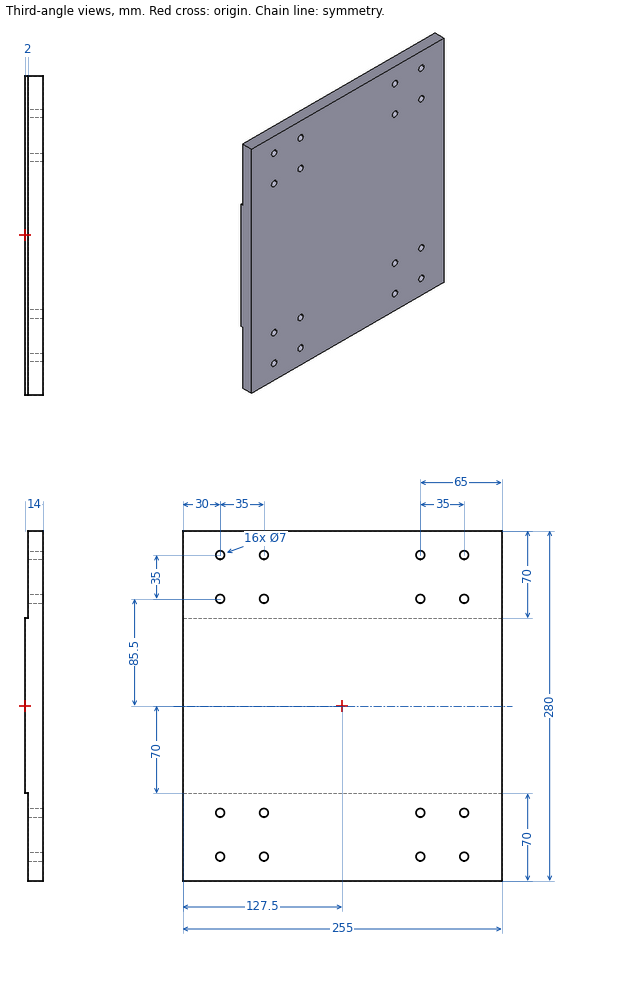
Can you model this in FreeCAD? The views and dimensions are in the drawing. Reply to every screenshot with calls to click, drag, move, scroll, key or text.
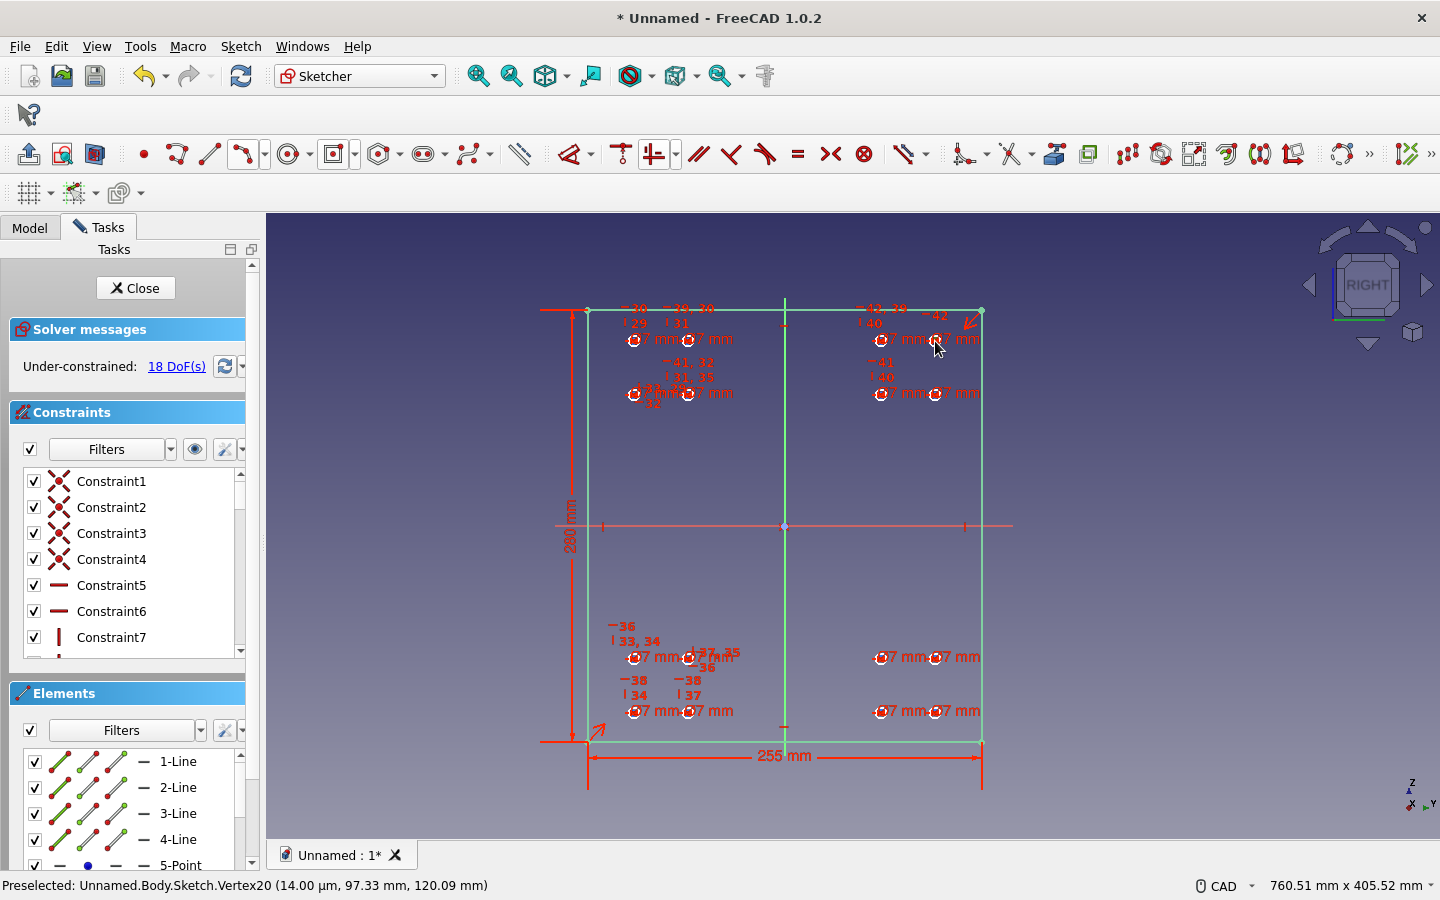
click(935, 395)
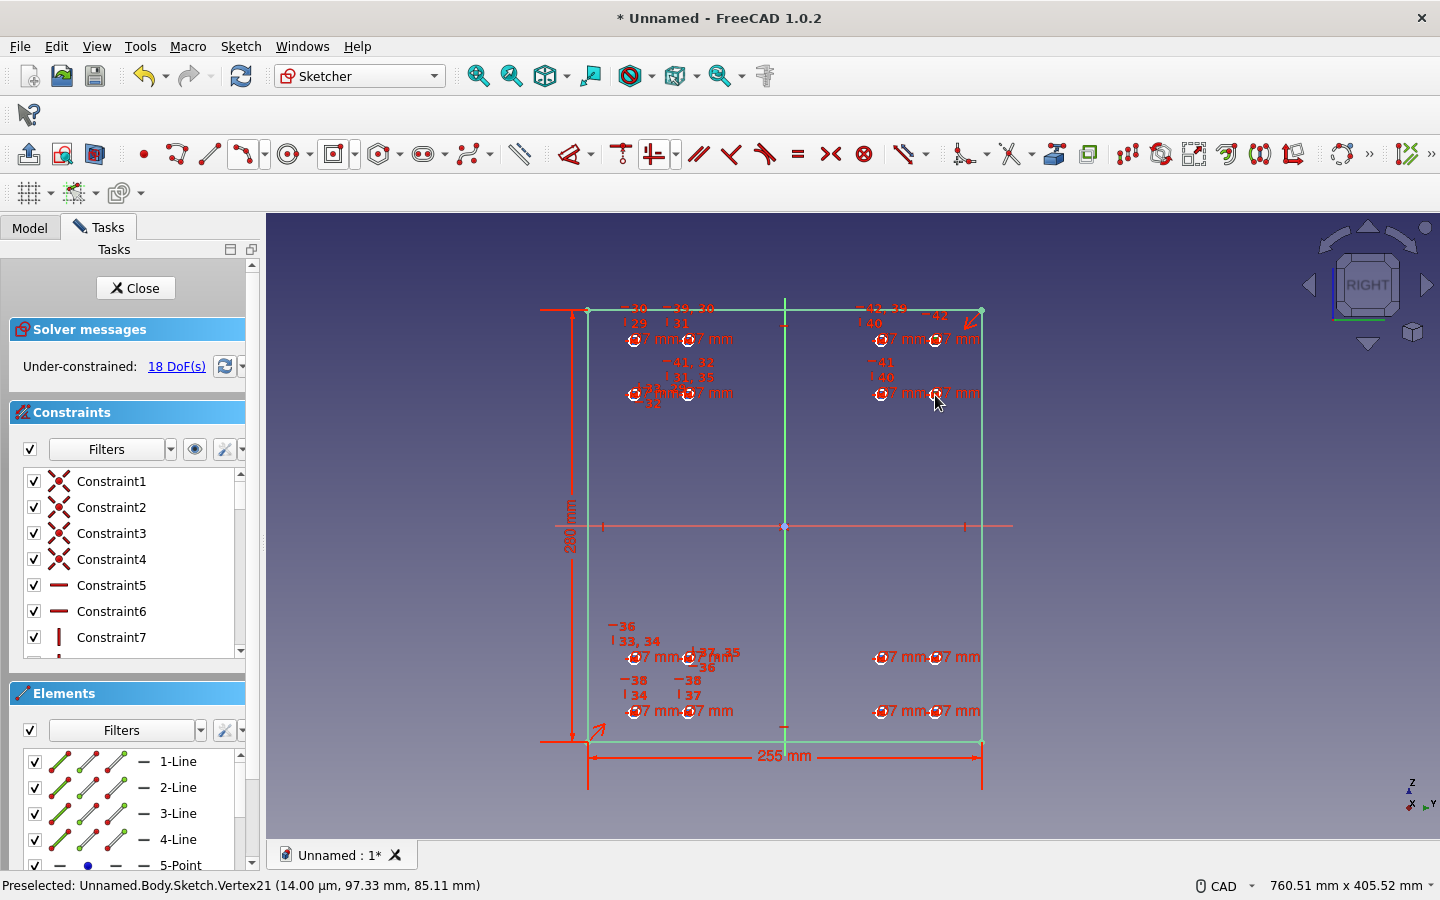
click(676, 154)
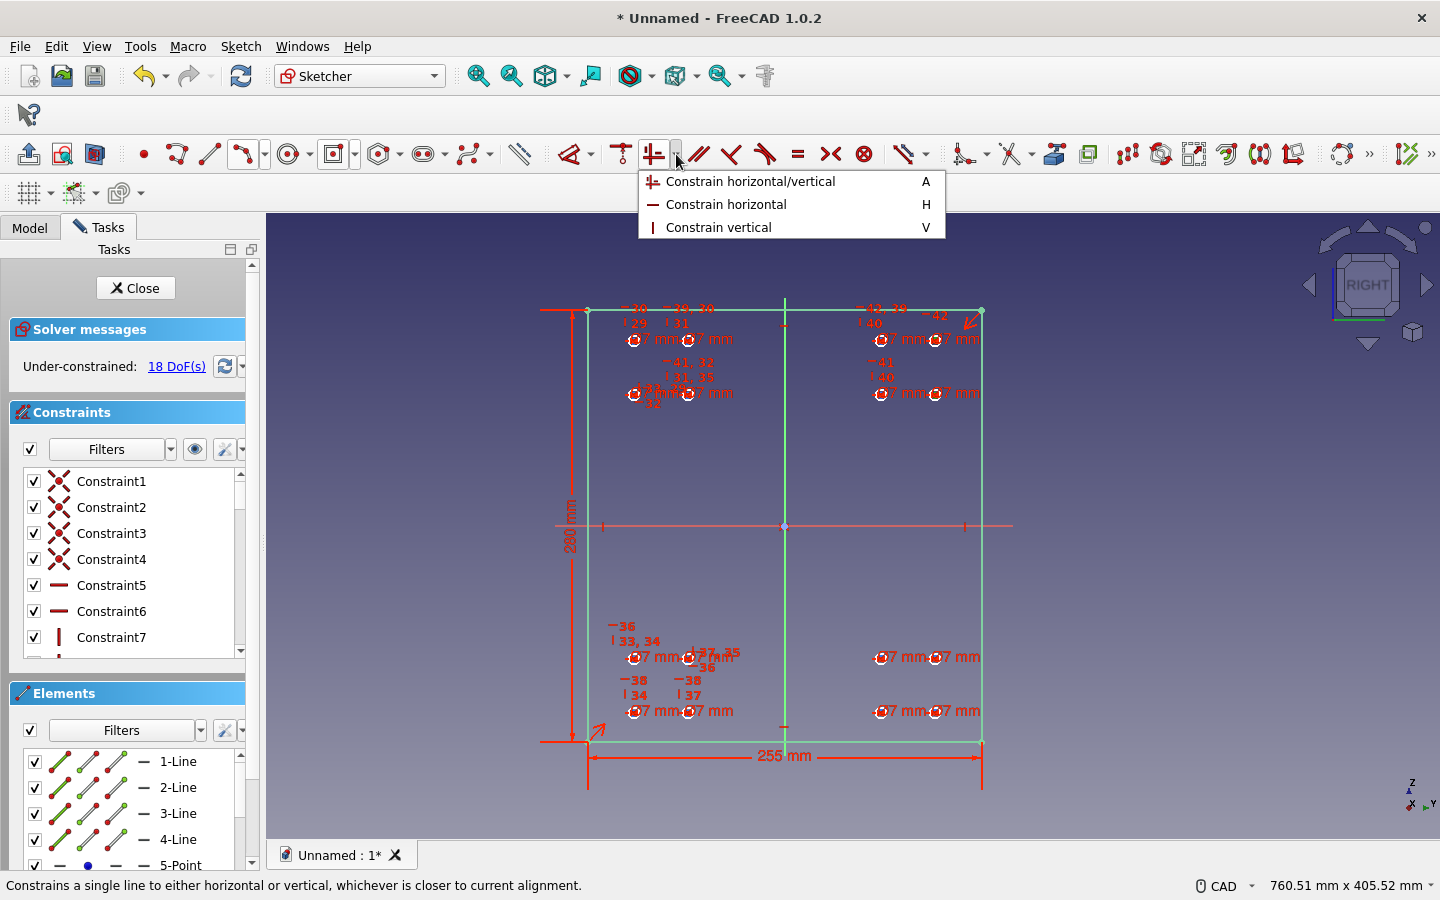
click(792, 228)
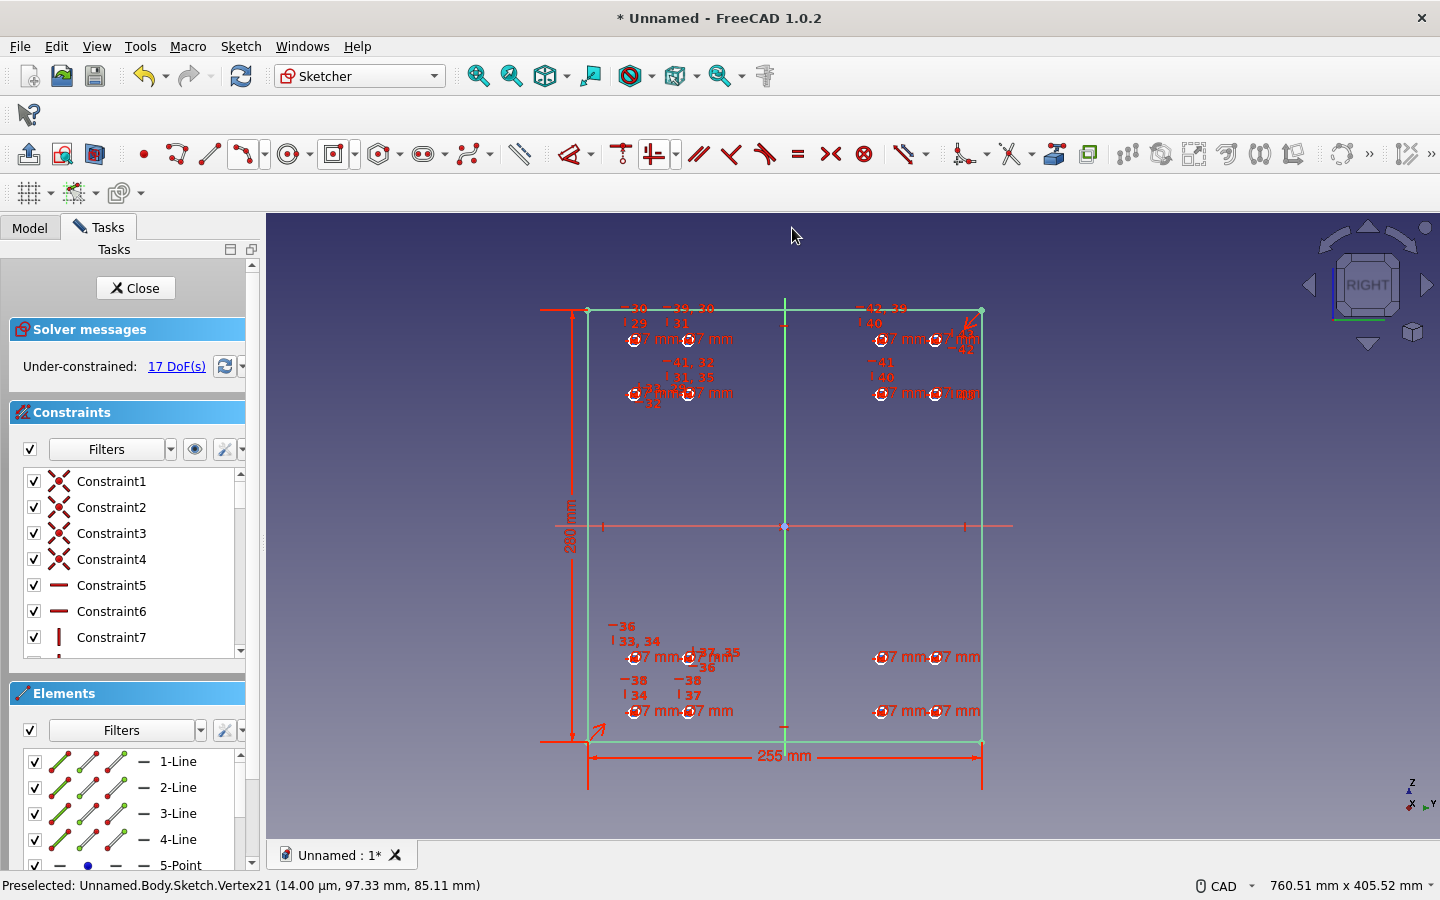
click(881, 395)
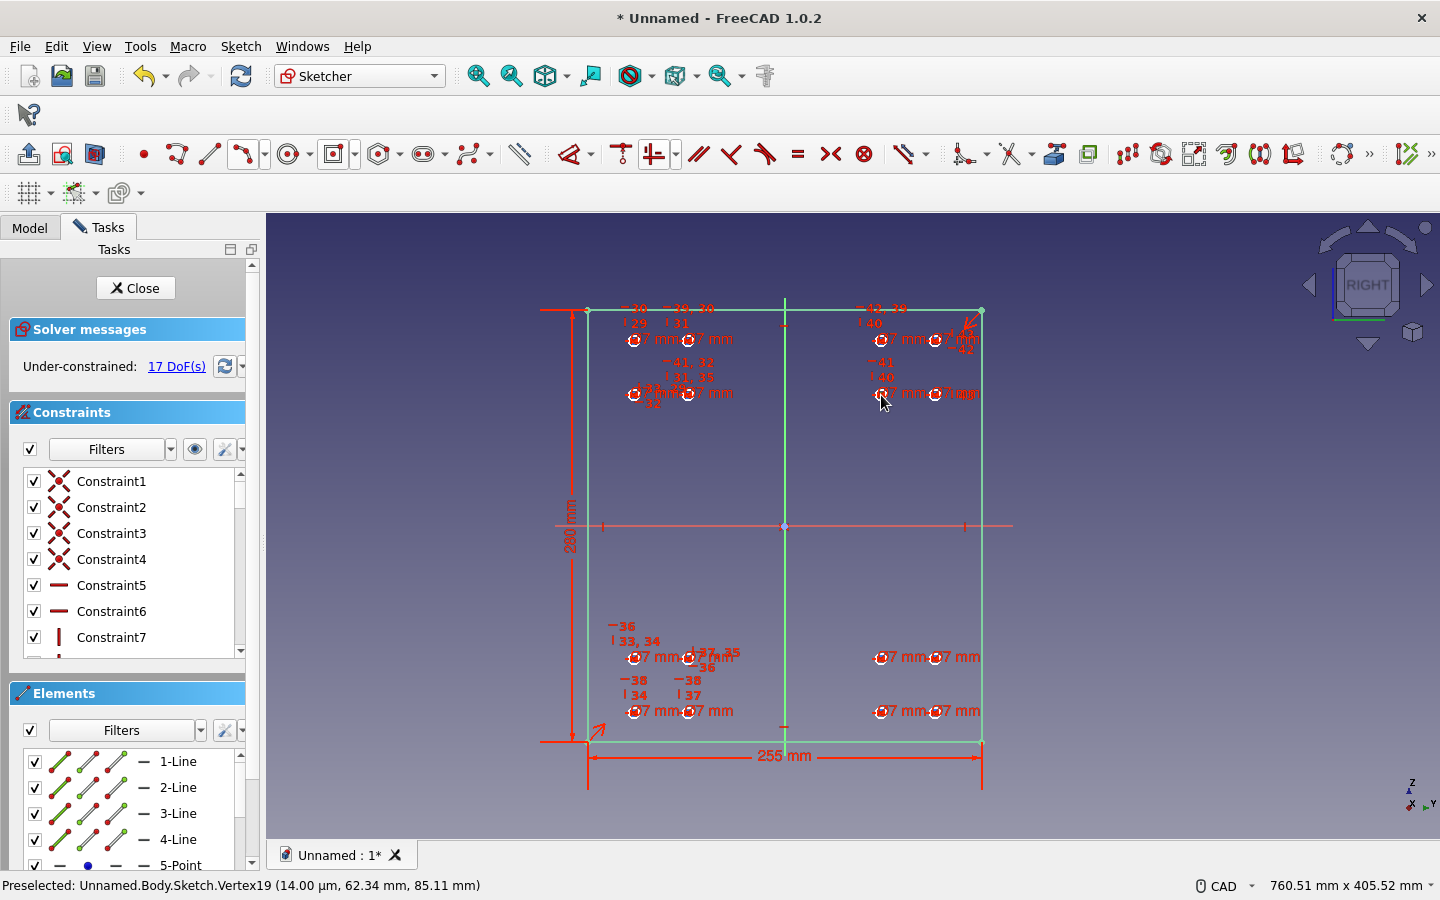
click(935, 395)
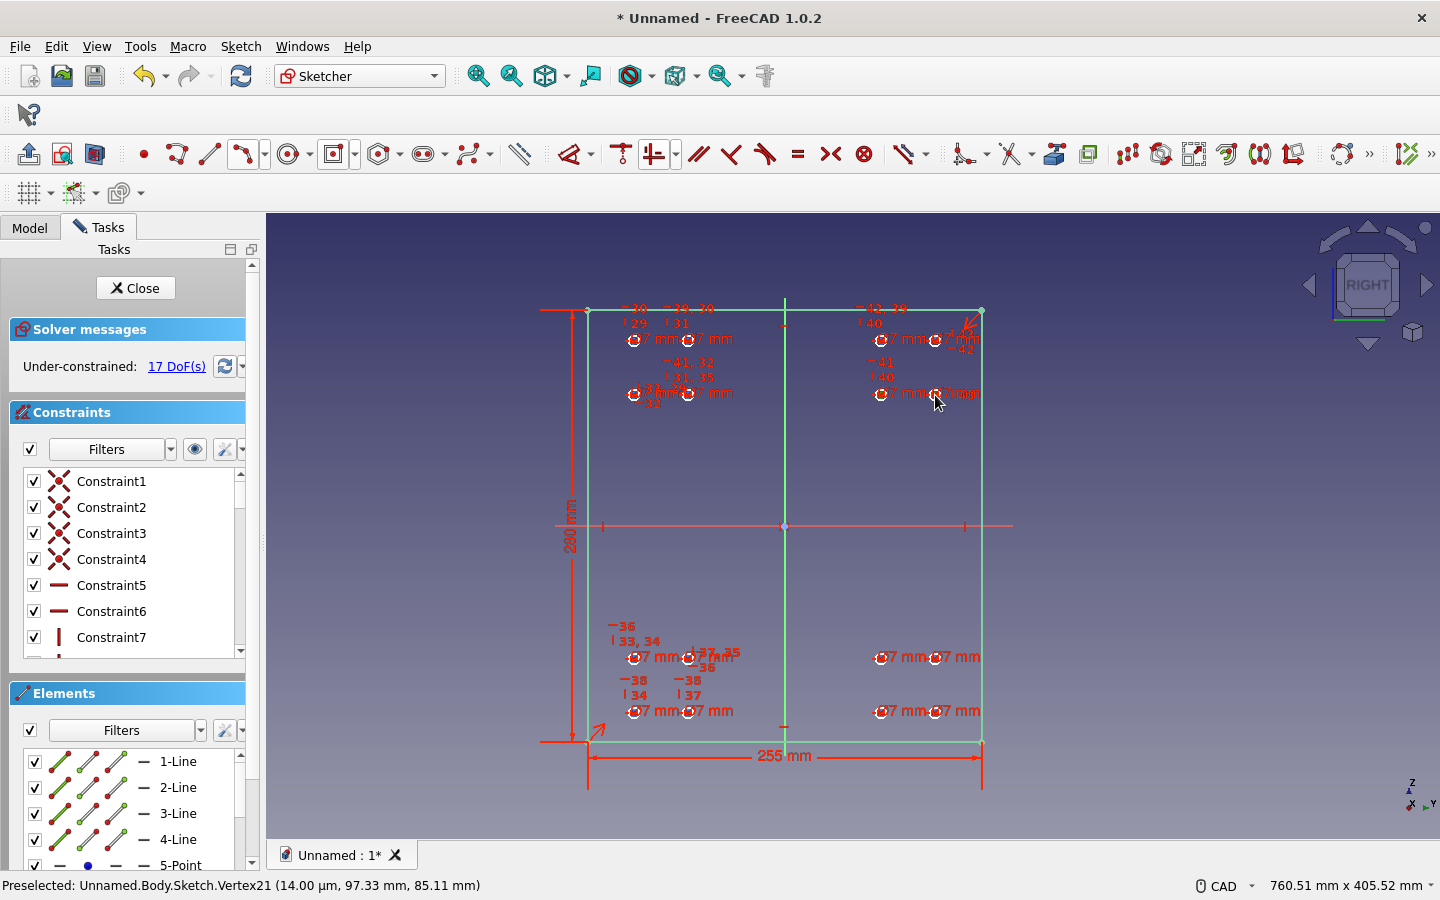
click(676, 154)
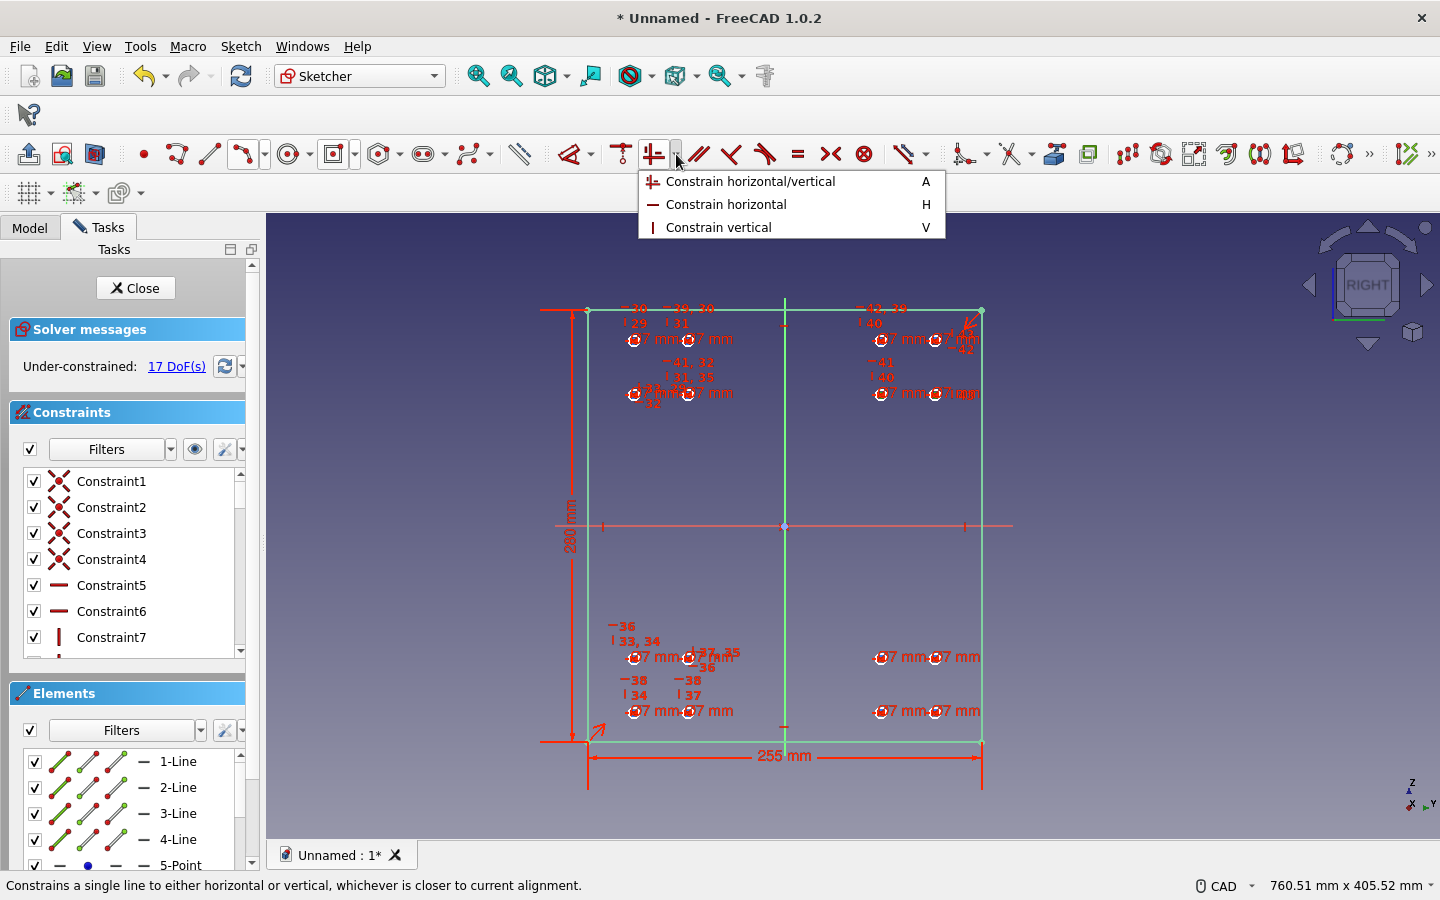
click(792, 204)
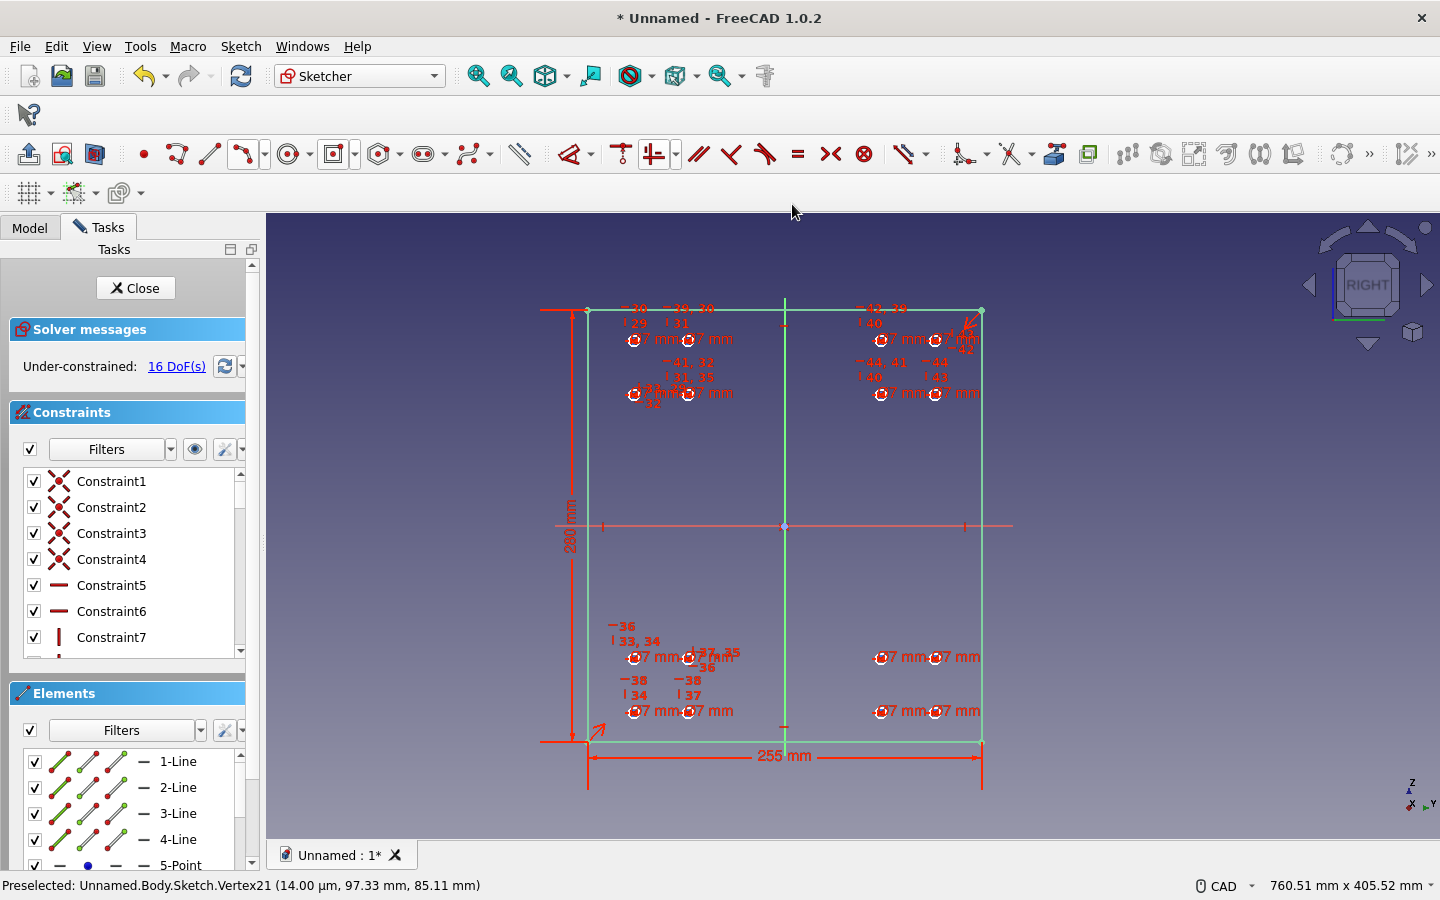
click(688, 659)